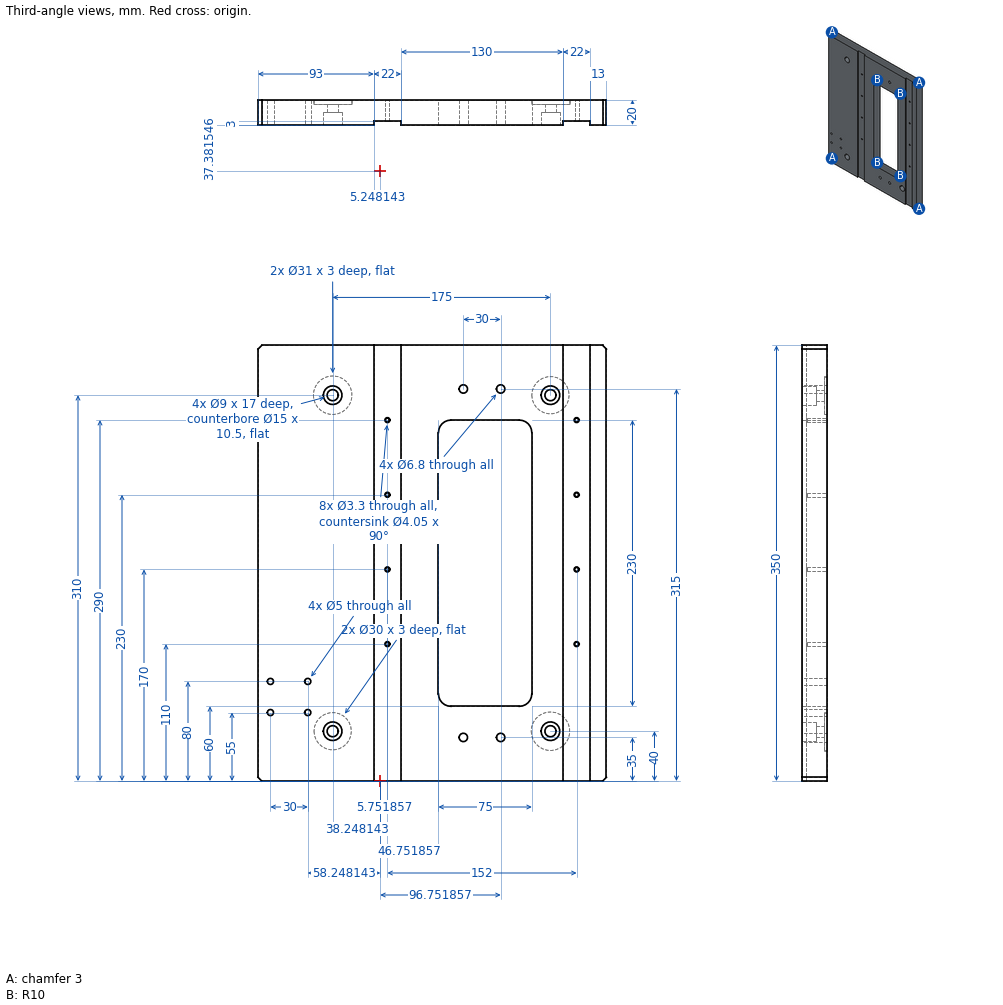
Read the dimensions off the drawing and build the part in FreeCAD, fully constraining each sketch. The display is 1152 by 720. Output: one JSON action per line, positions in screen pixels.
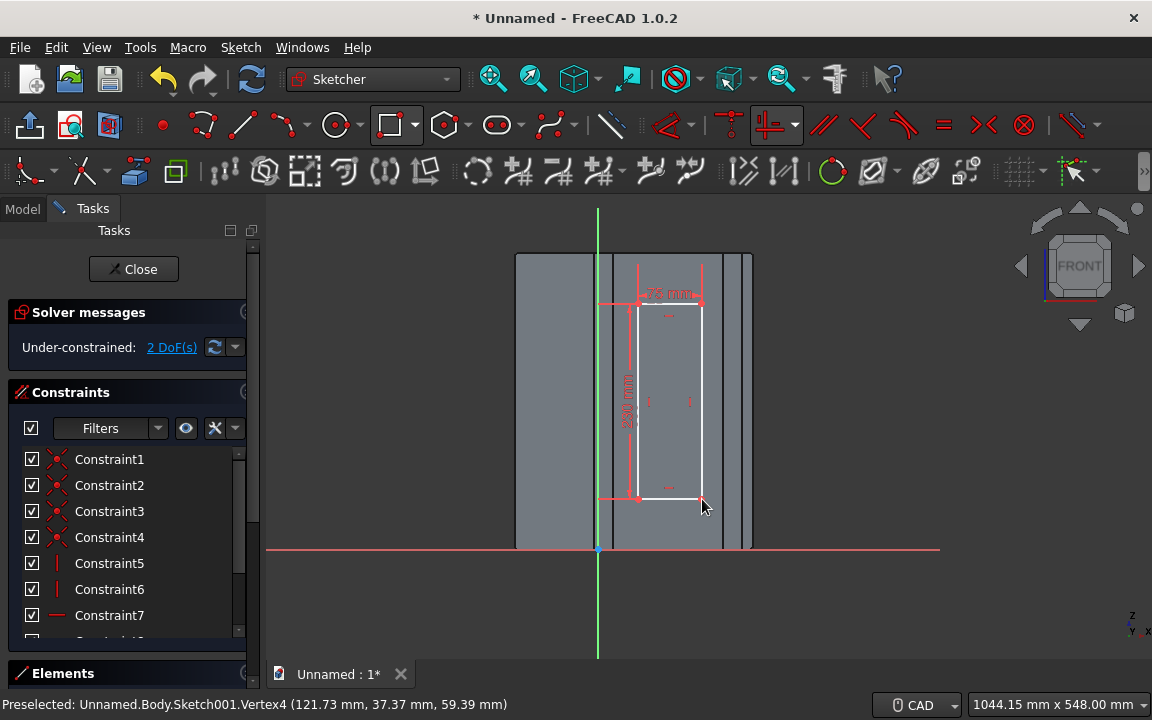
{"action": "left_click", "coordinate": [666, 126]}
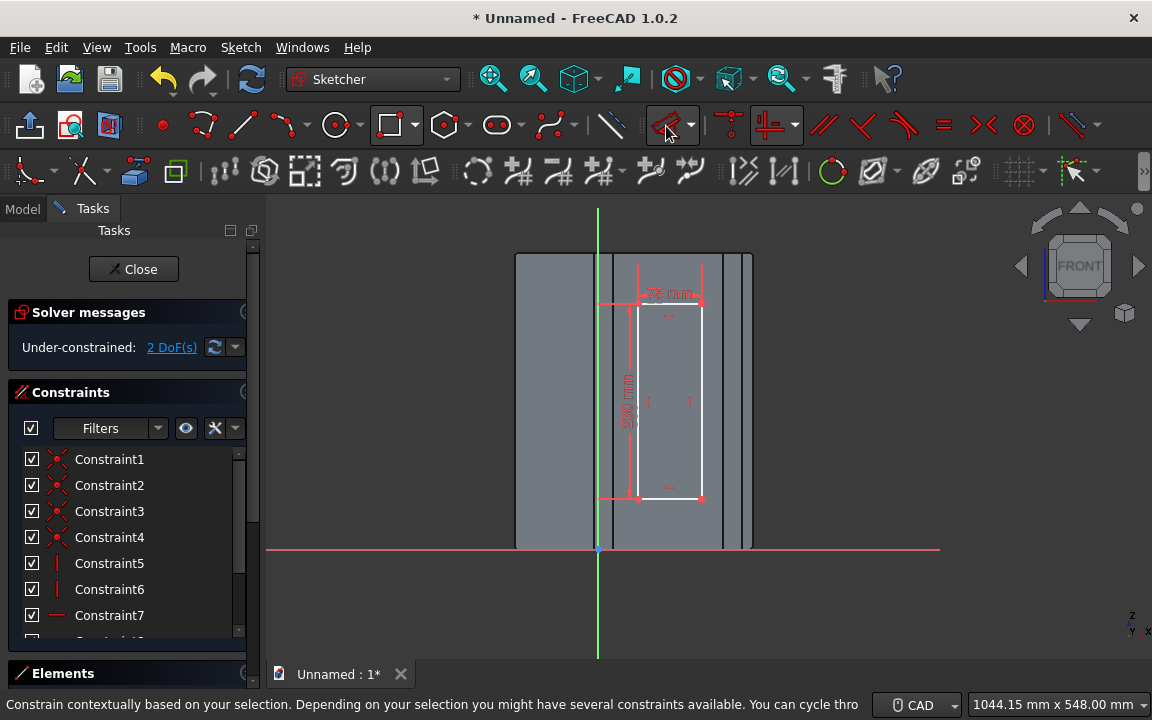
{"action": "left_click", "coordinate": [638, 499]}
{"action": "left_click", "coordinate": [564, 524]}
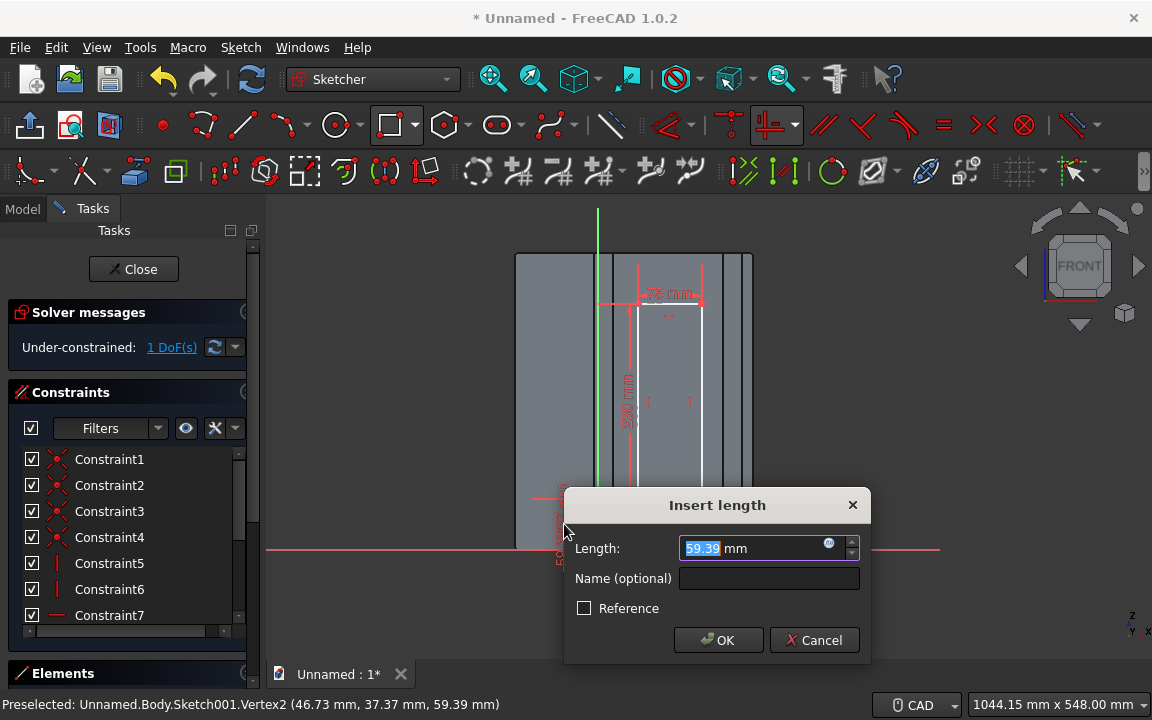
{"action": "type", "text": "60"}
{"action": "key", "text": "Return"}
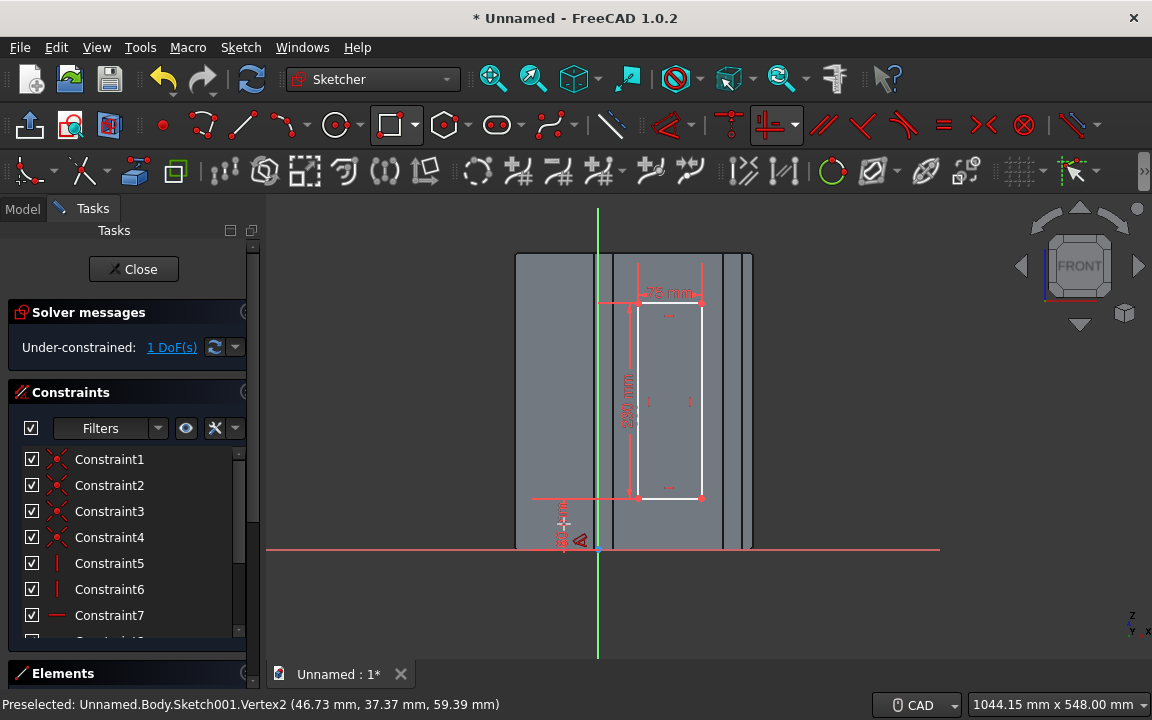
{"action": "left_click", "coordinate": [638, 303]}
{"action": "left_click", "coordinate": [618, 584]}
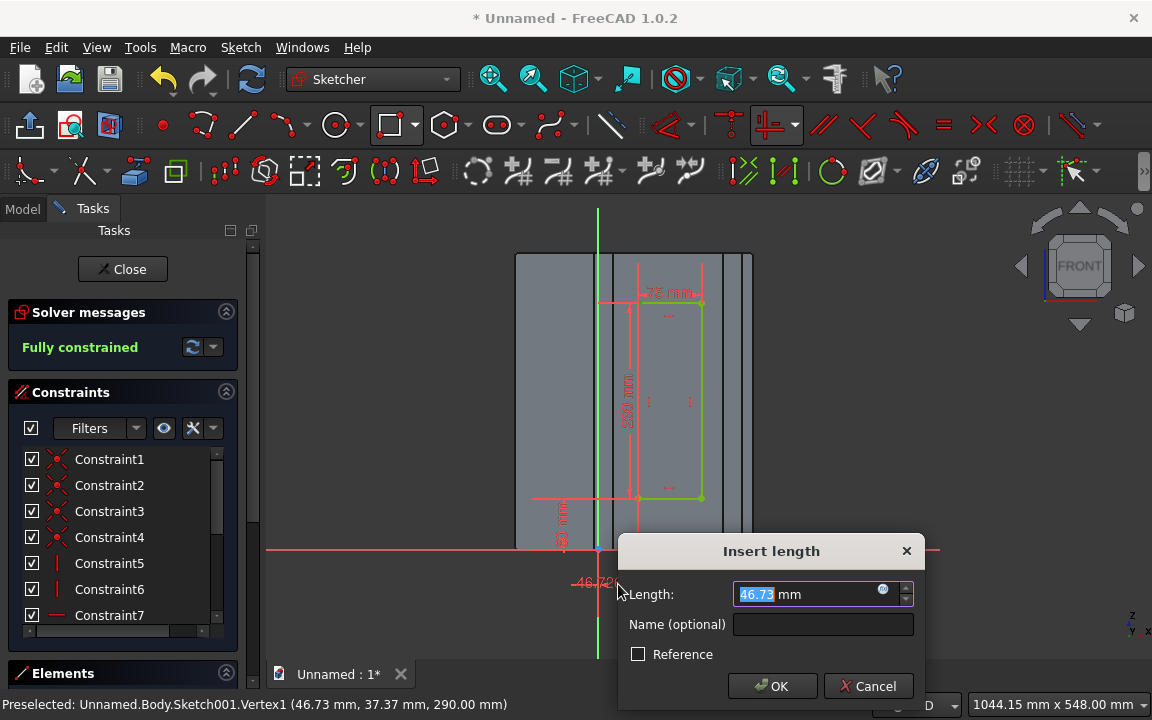
{"action": "type", "text": "46.751857"}
{"action": "key", "text": "Return"}
{"action": "key", "text": "Escape"}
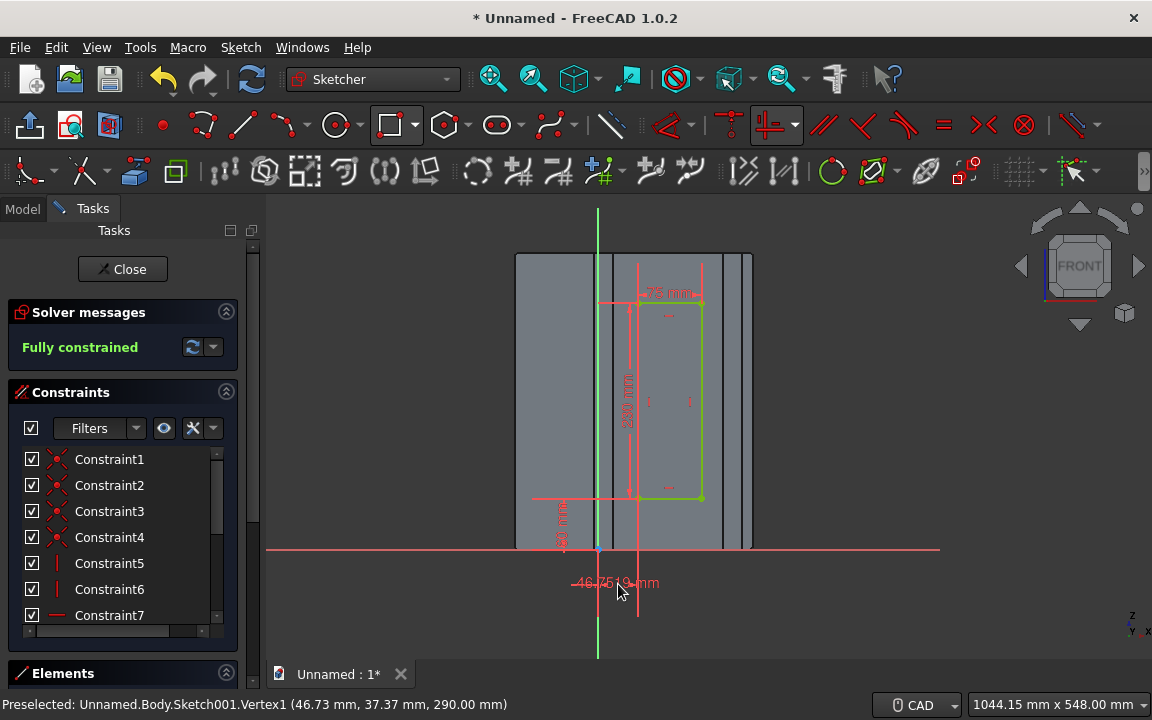
{"action": "left_click", "coordinate": [123, 269]}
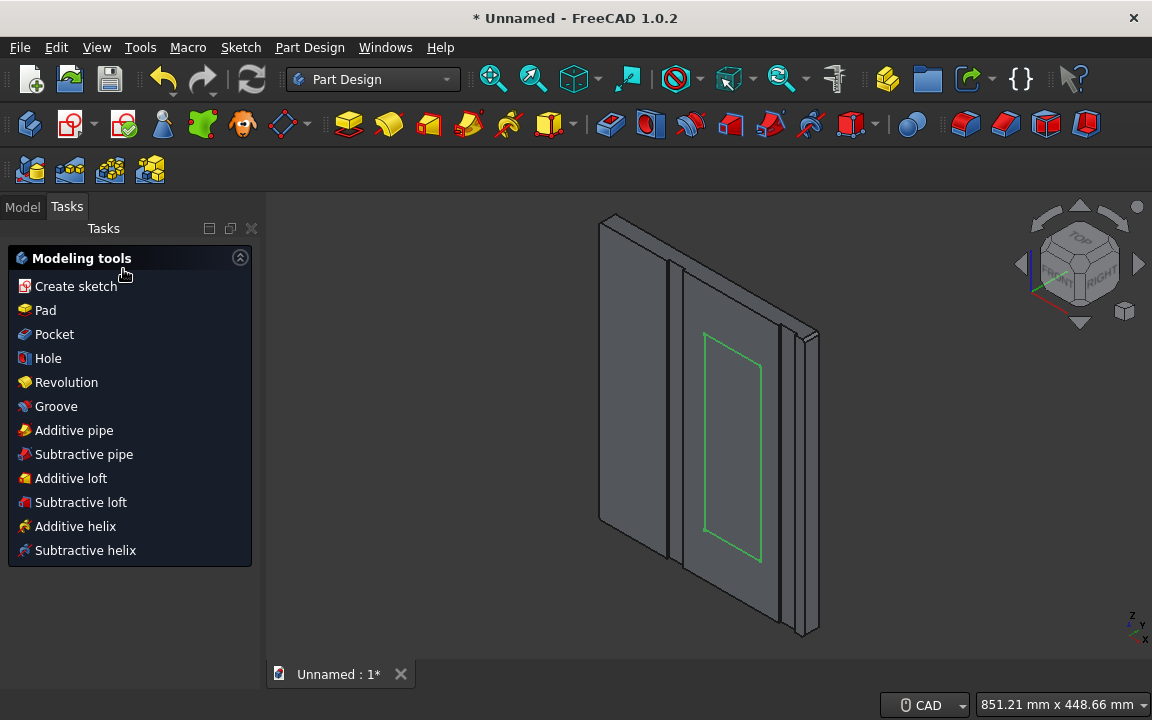
{"action": "left_click", "coordinate": [612, 124]}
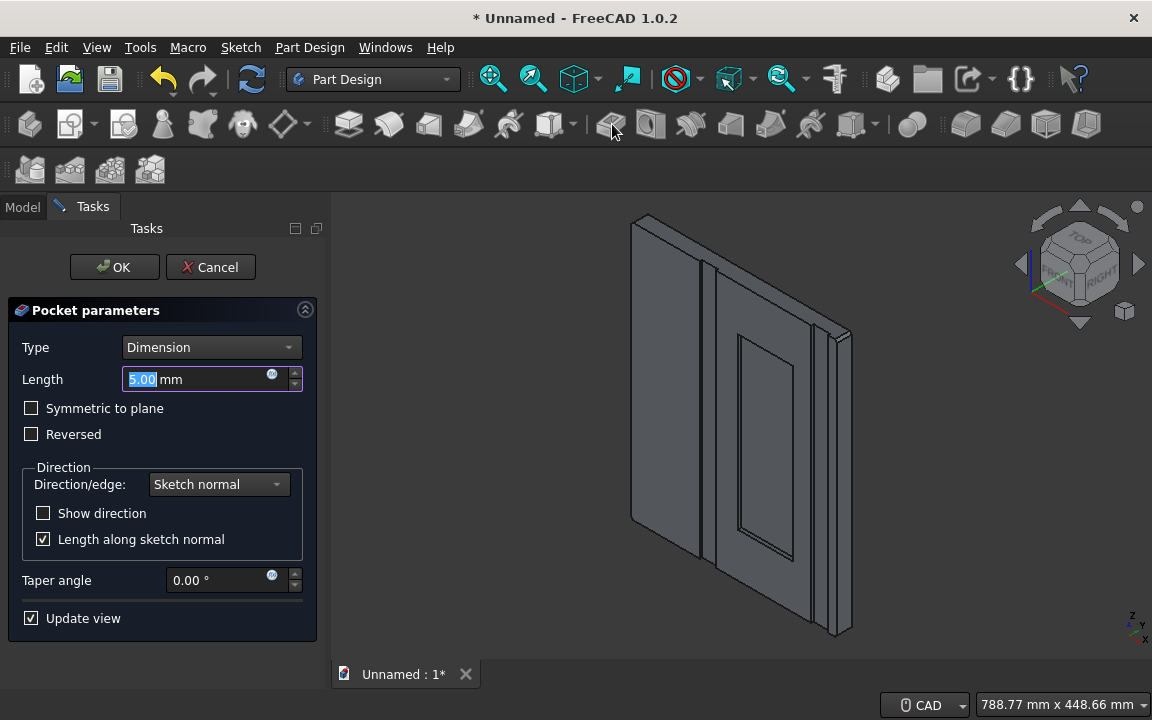
{"action": "left_click", "coordinate": [212, 348]}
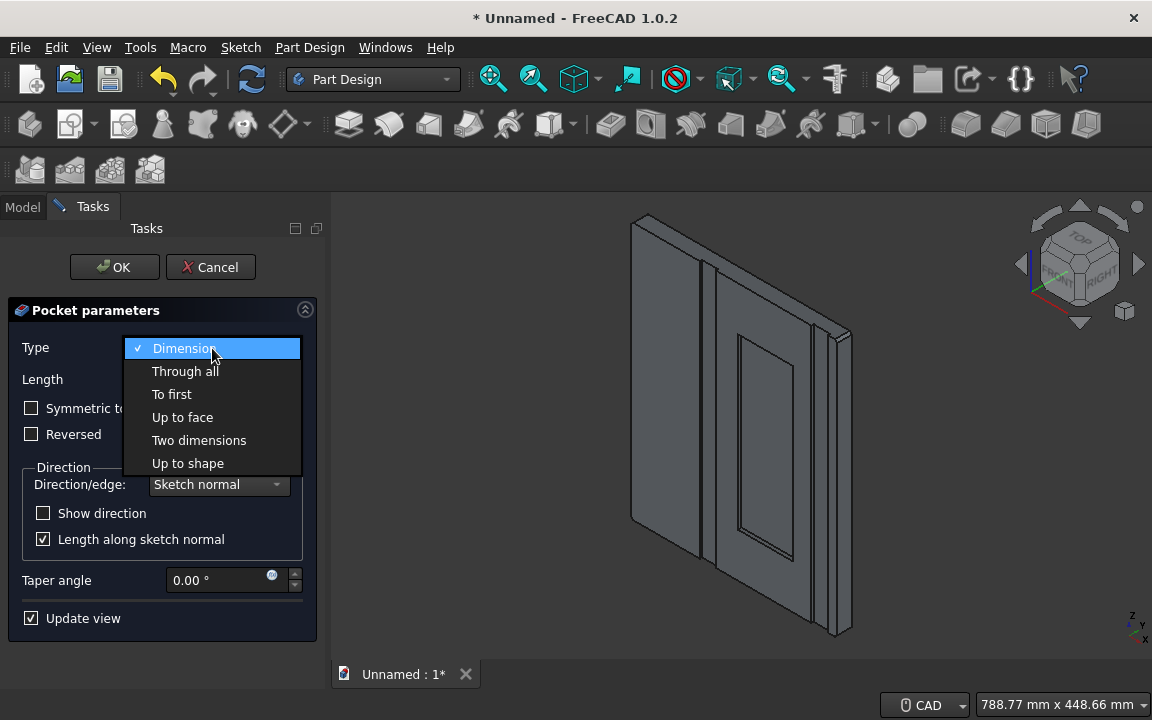
{"action": "left_click", "coordinate": [212, 372]}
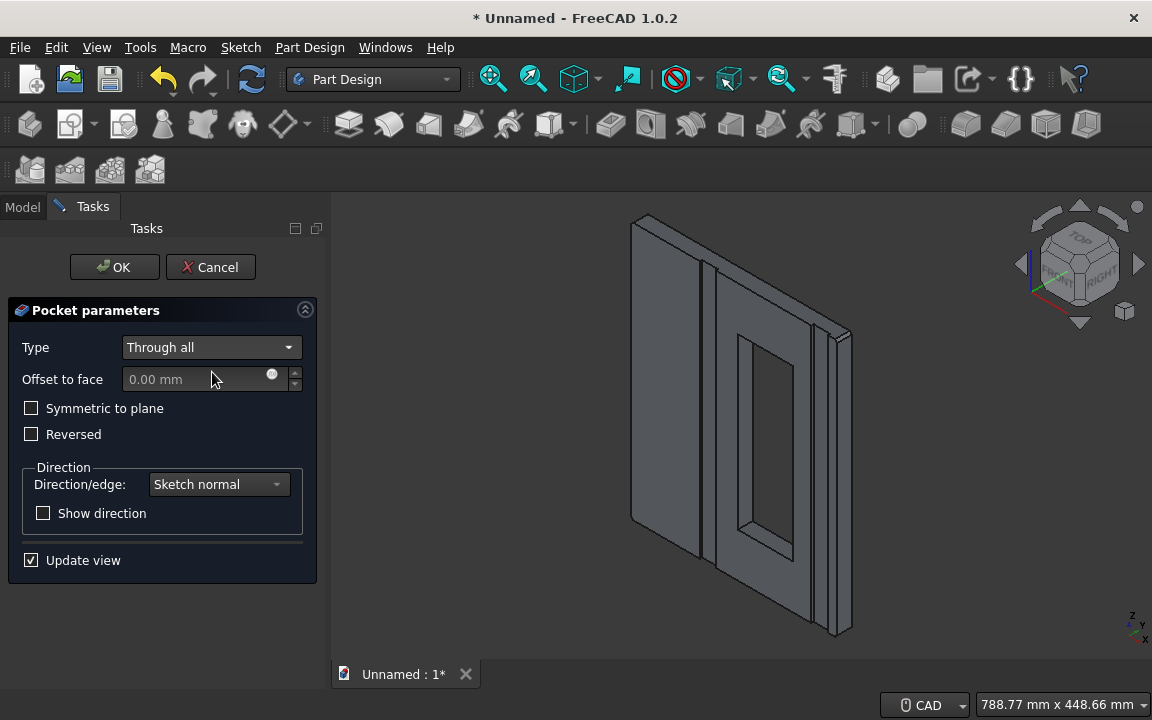
{"action": "left_click", "coordinate": [115, 267]}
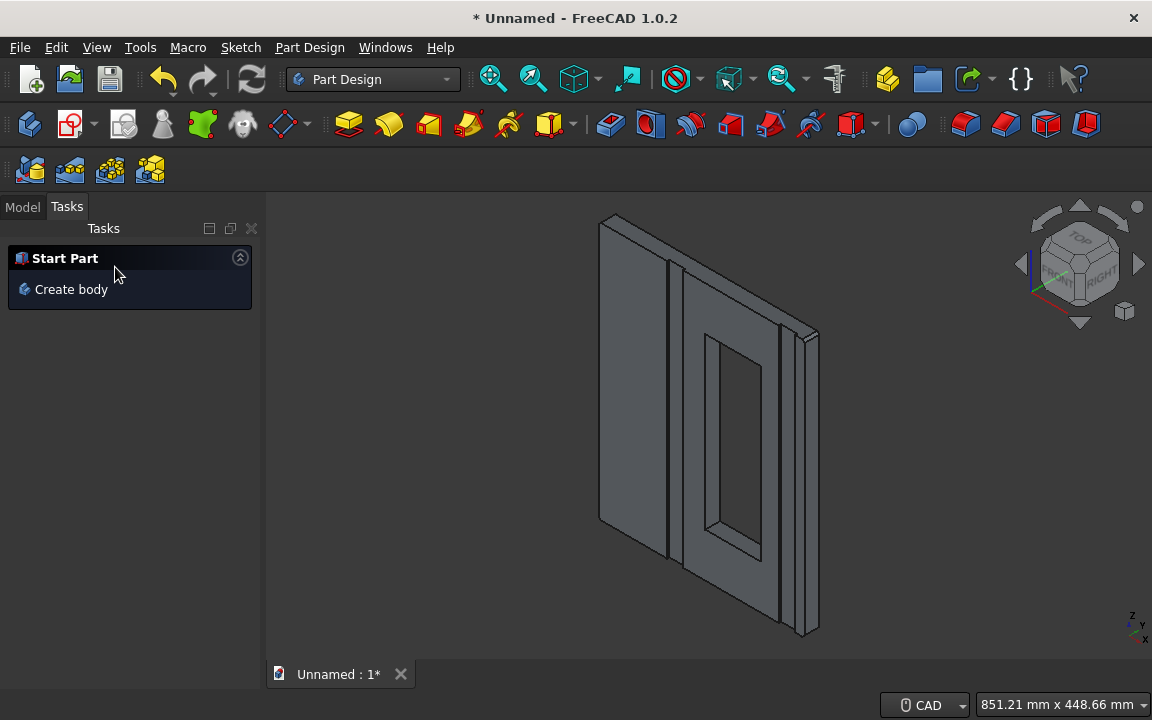
{"action": "scroll", "coordinate": [713, 524], "scroll_direction": "up", "scroll_amount": 4}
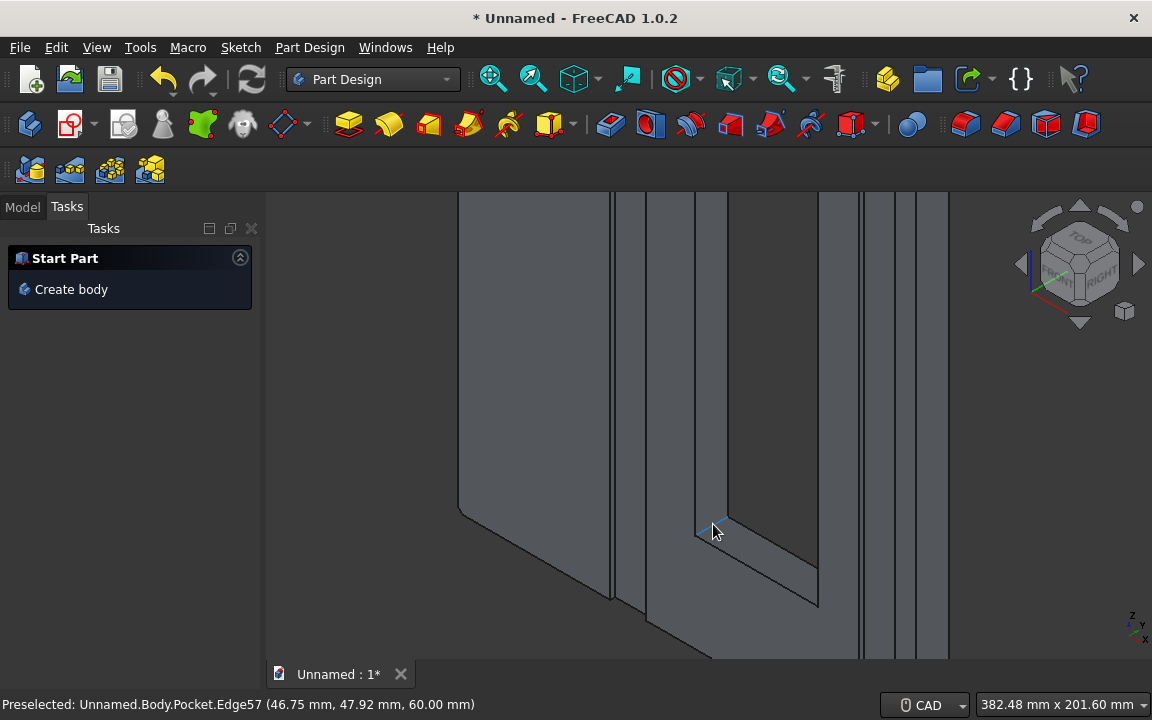
{"action": "left_click", "coordinate": [494, 80]}